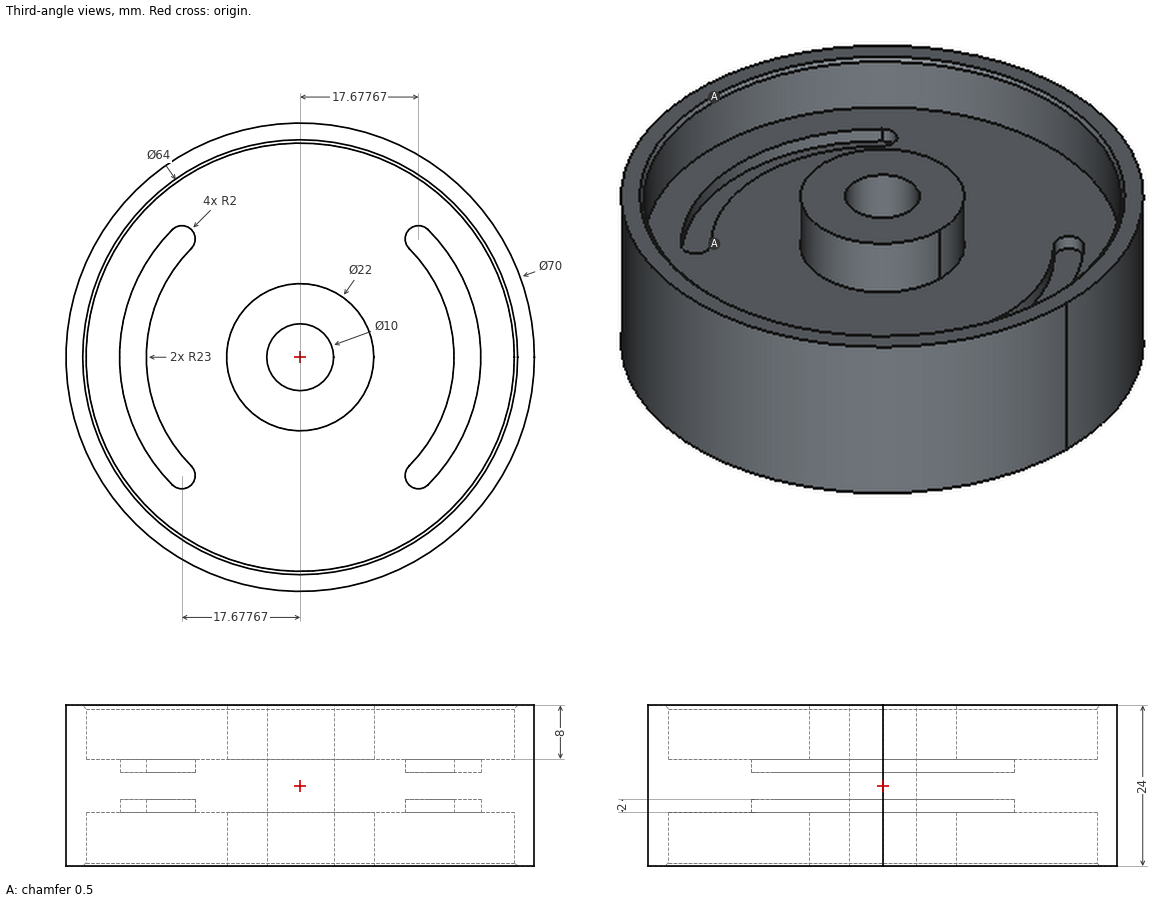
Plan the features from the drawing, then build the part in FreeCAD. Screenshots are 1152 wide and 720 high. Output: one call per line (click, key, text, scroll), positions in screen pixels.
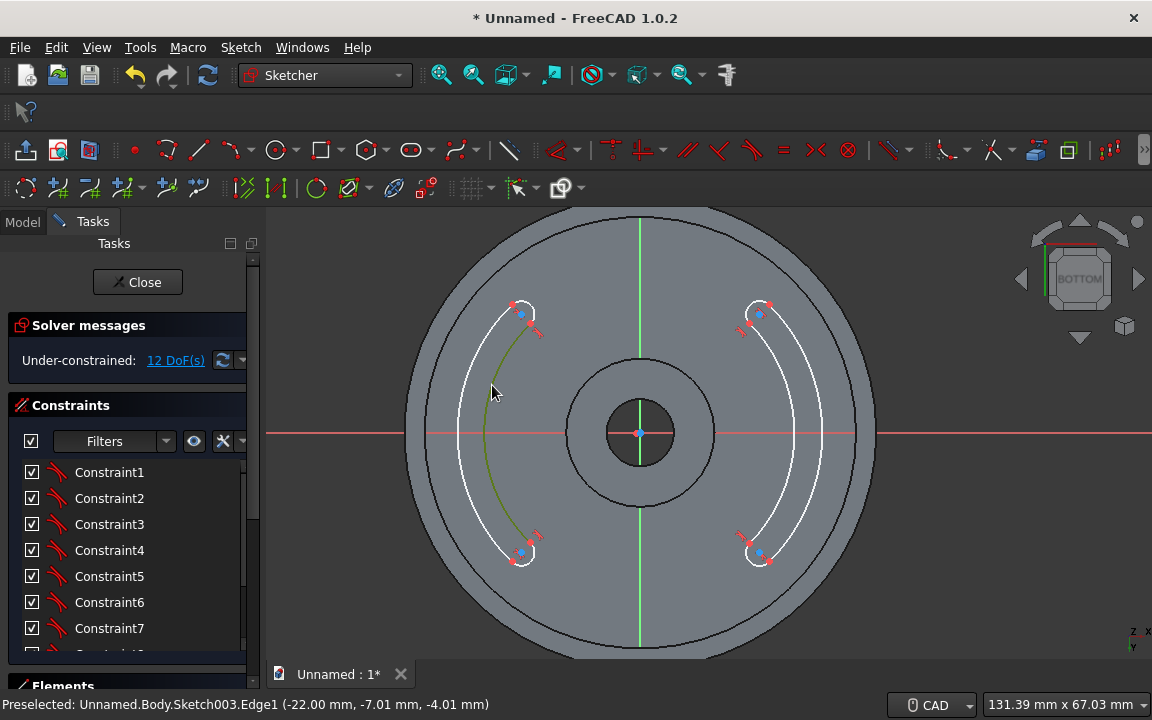
click(813, 490)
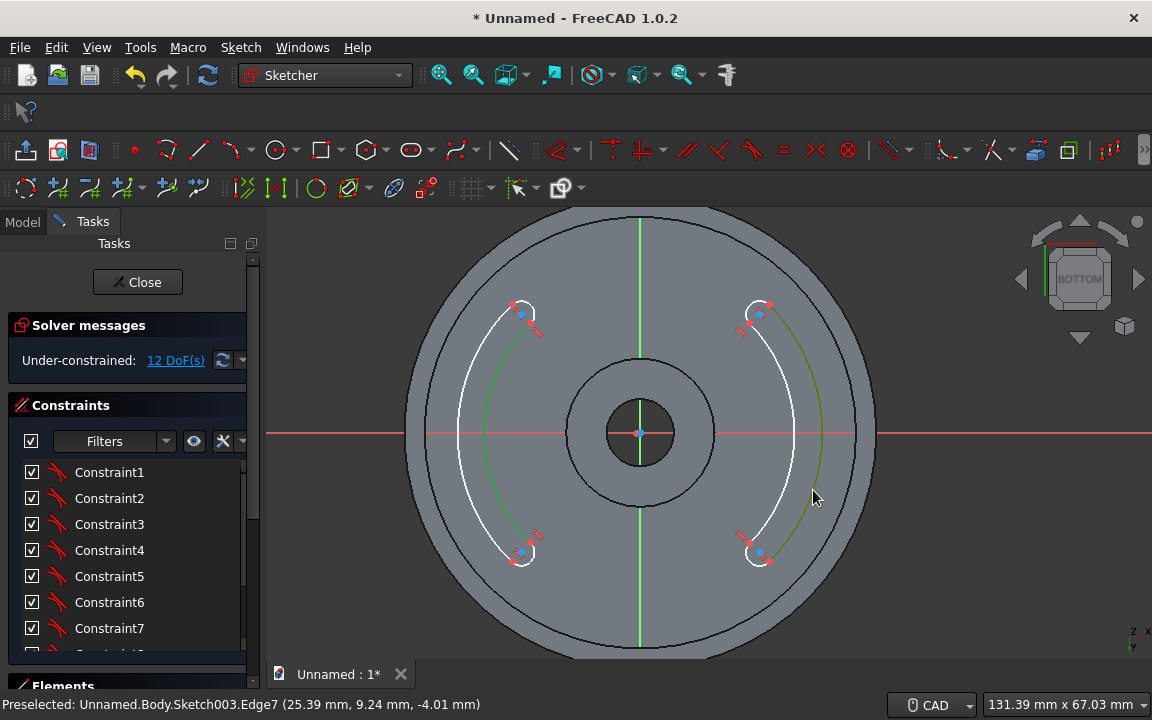
key(c)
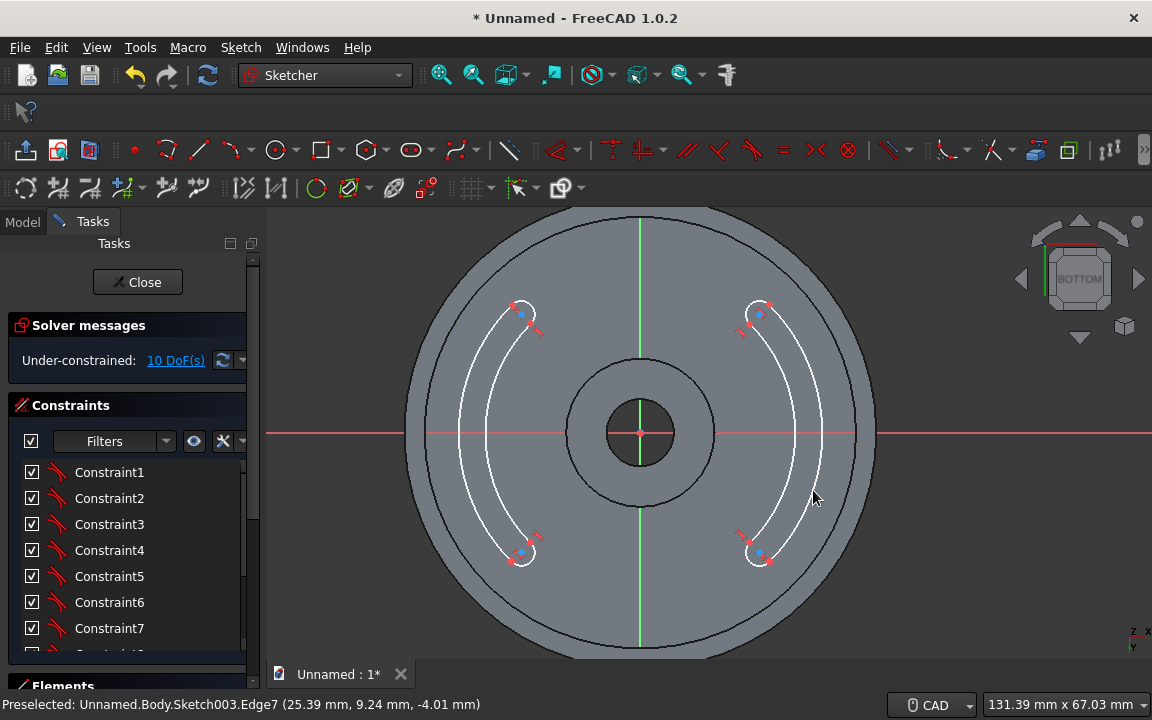
scroll(640, 433, up, 6)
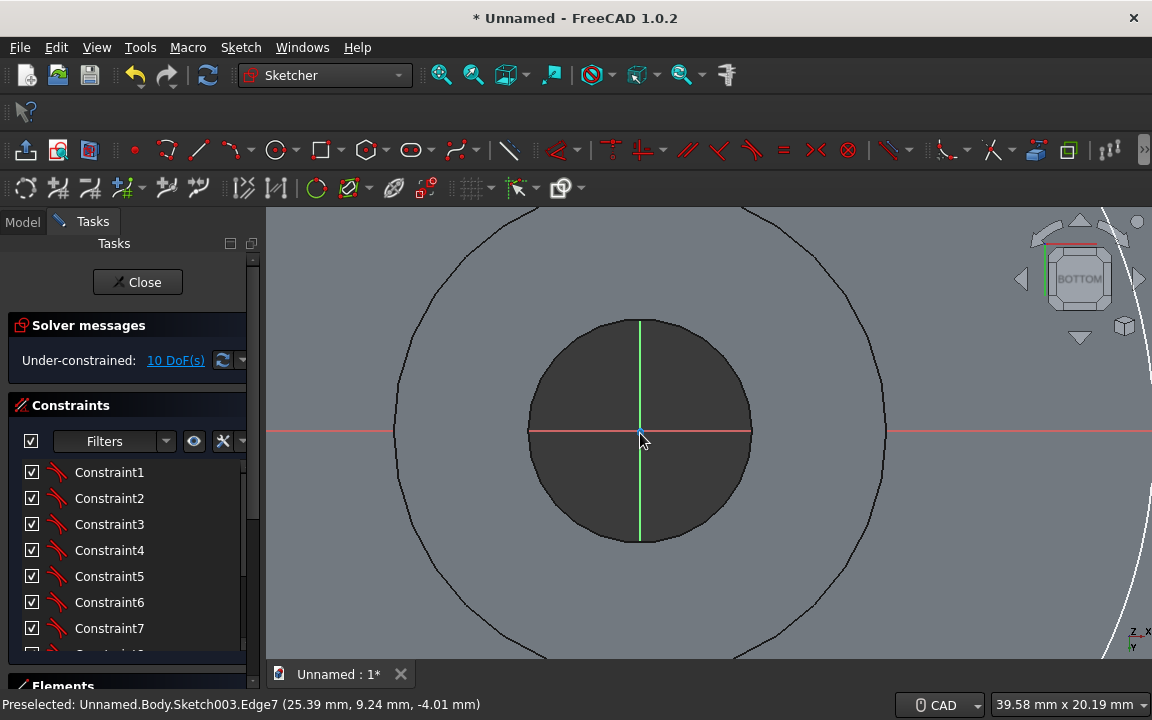
drag(630, 421, 651, 443)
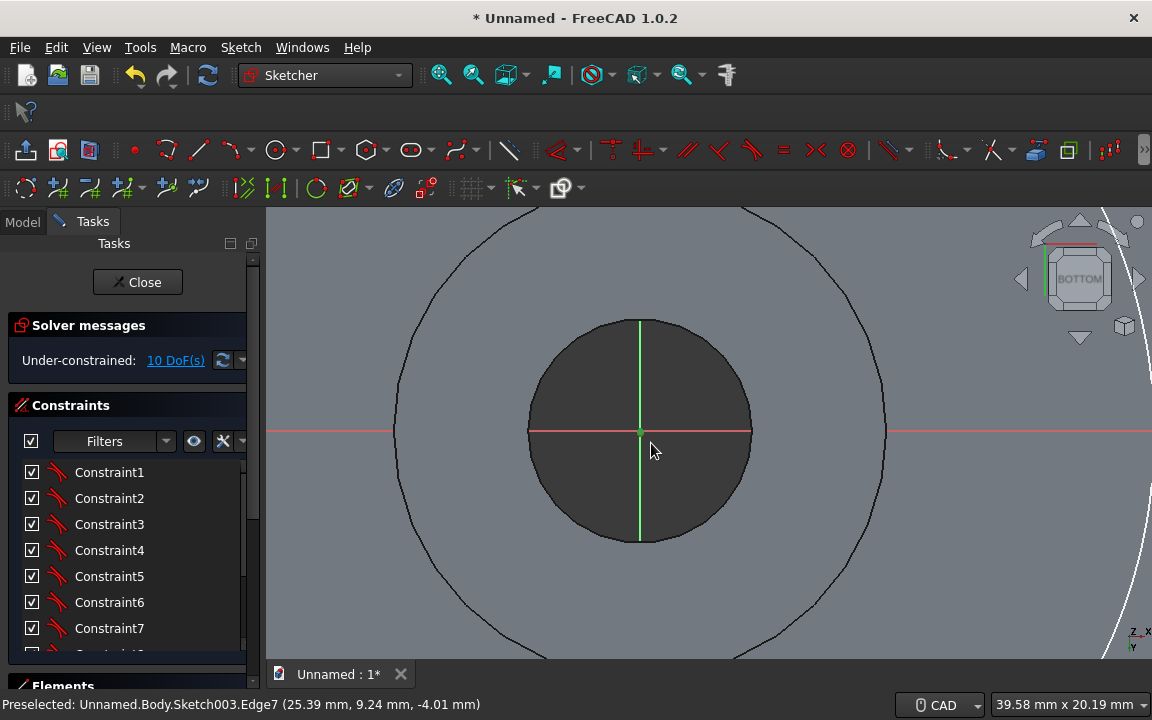
key(c)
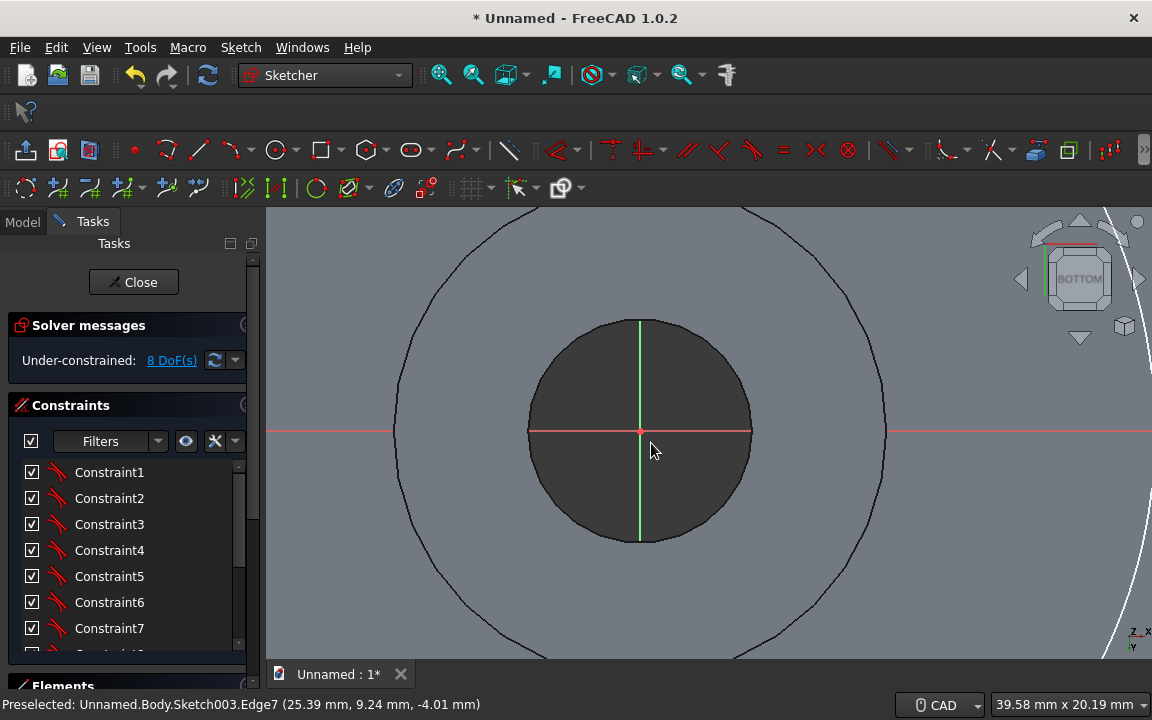
scroll(641, 434, down, 6)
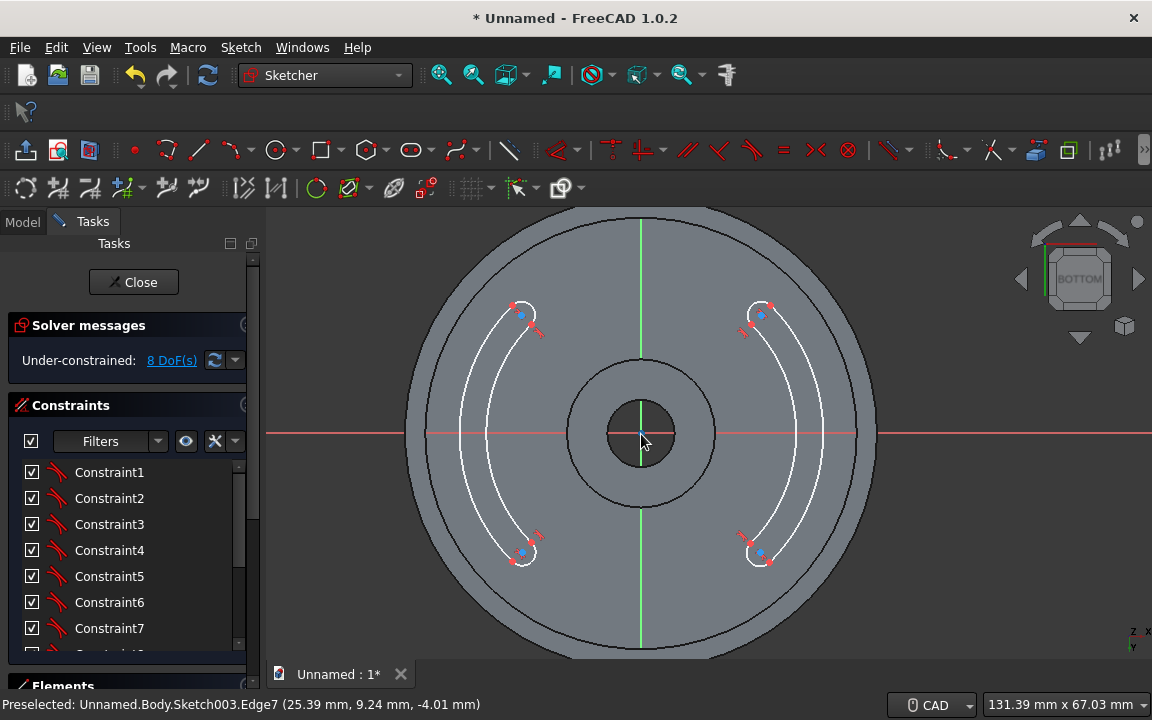
click(494, 386)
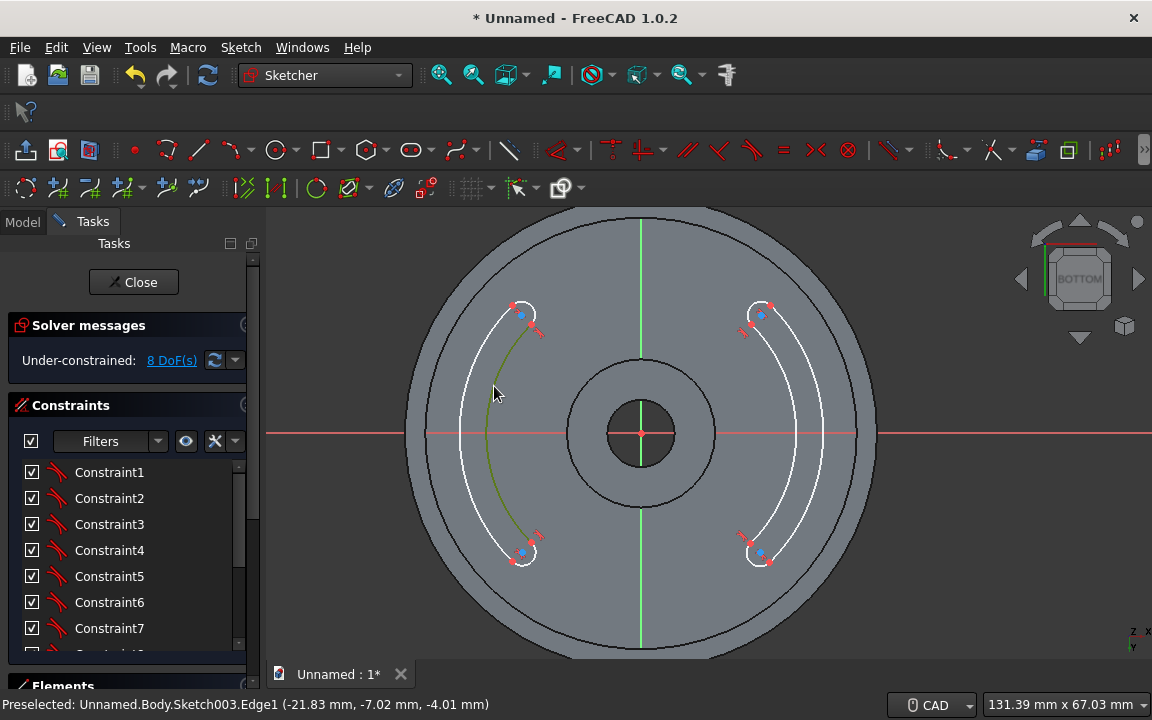
click(788, 482)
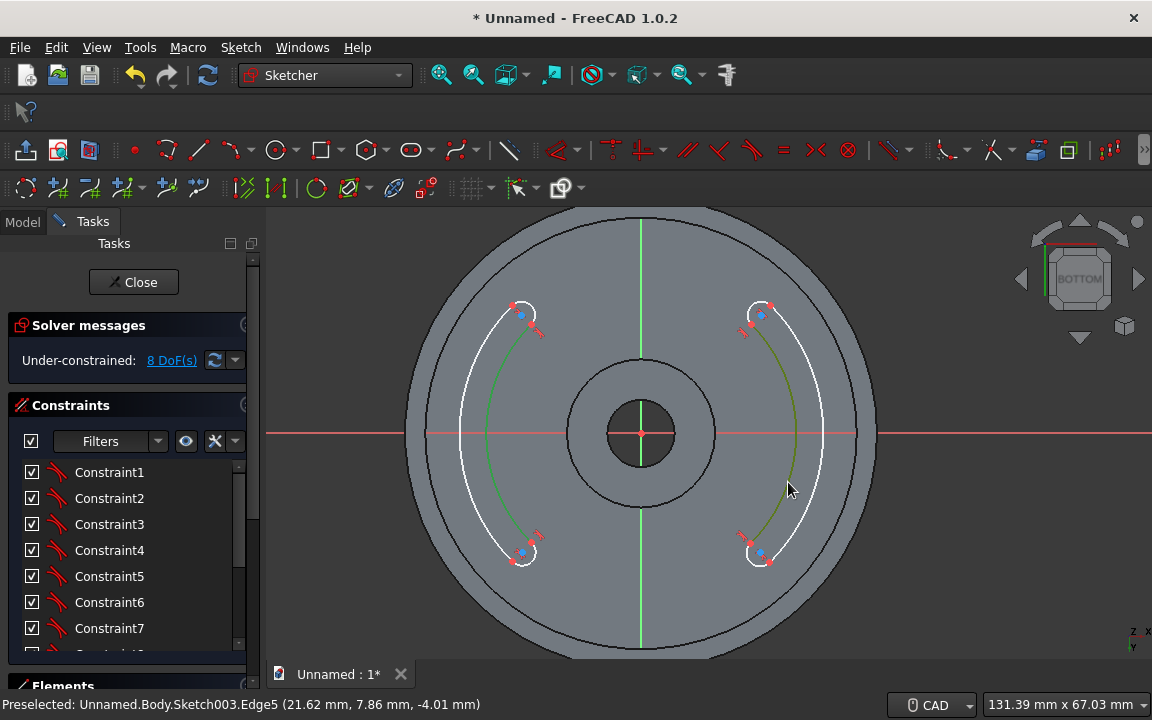
key(e)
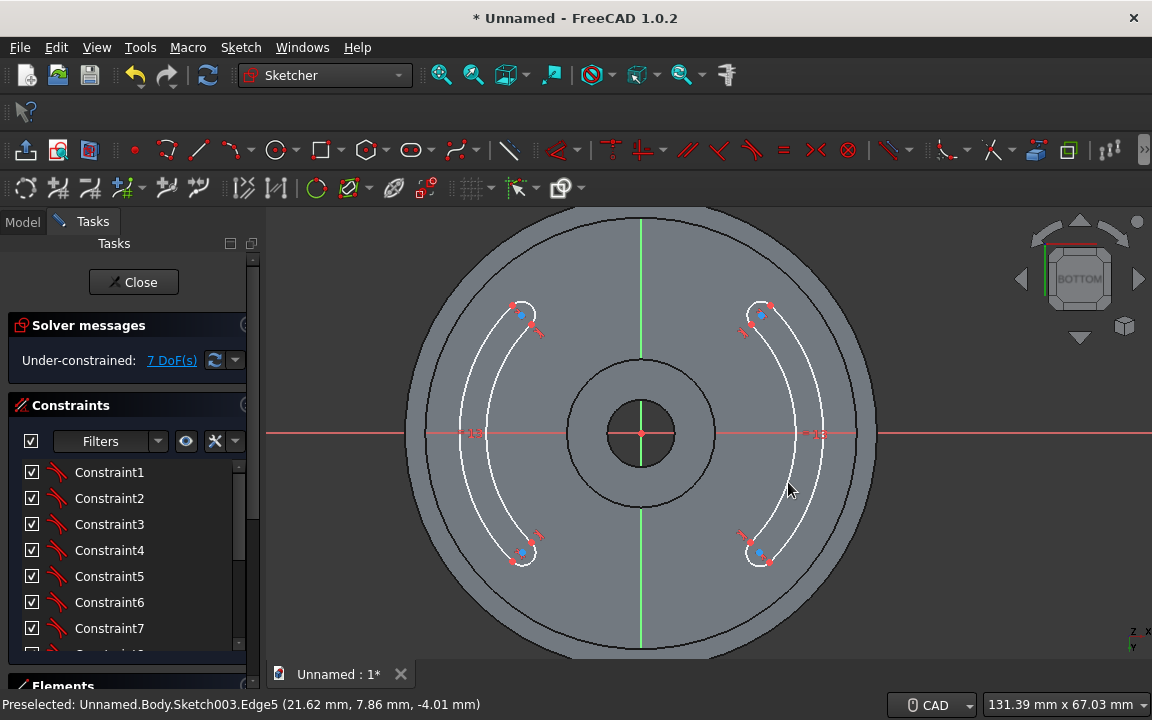
click(535, 313)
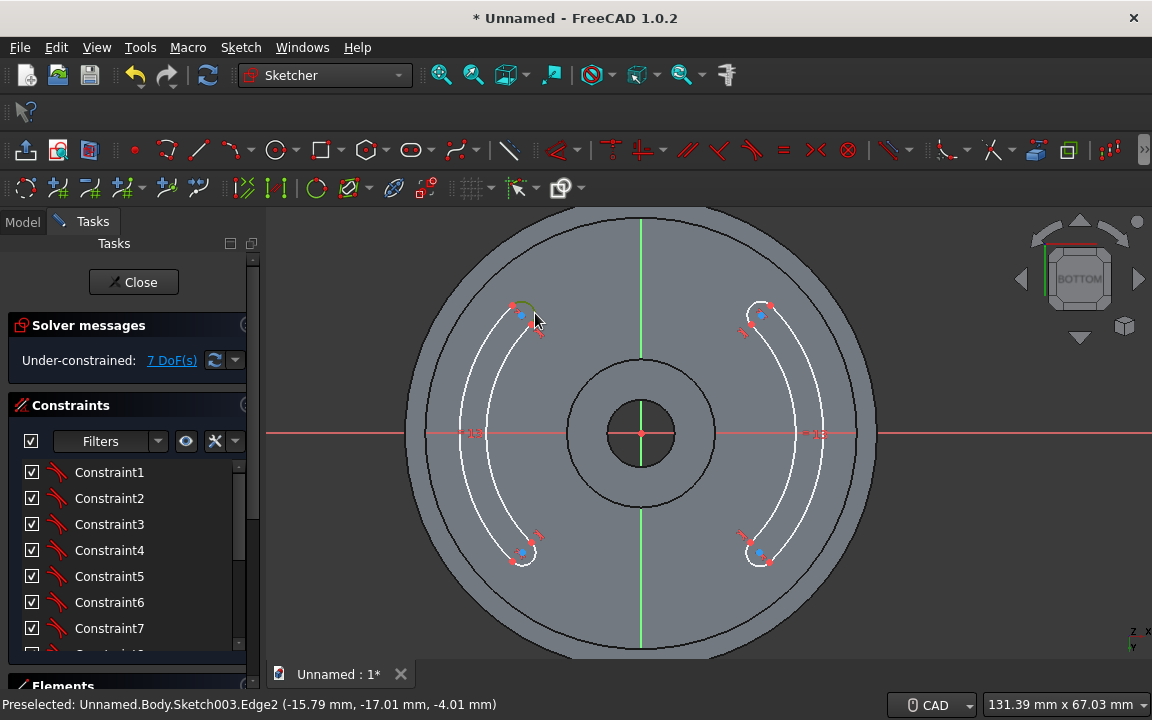
click(746, 555)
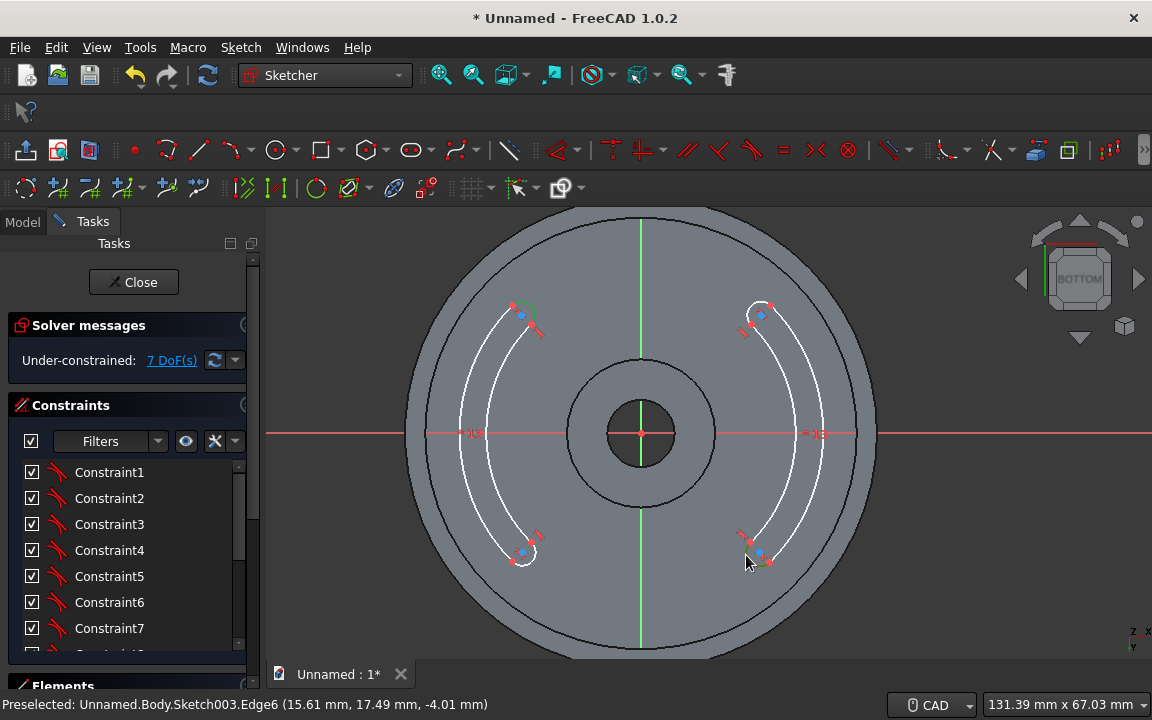
click(784, 150)